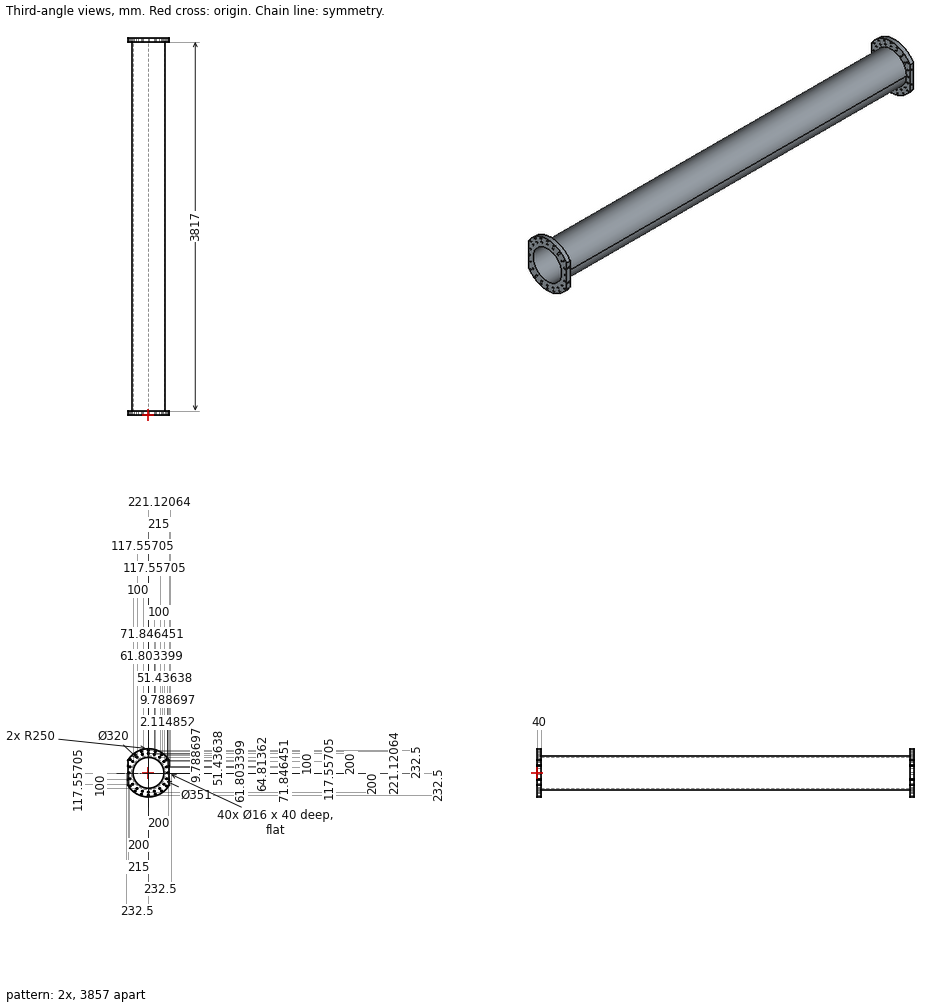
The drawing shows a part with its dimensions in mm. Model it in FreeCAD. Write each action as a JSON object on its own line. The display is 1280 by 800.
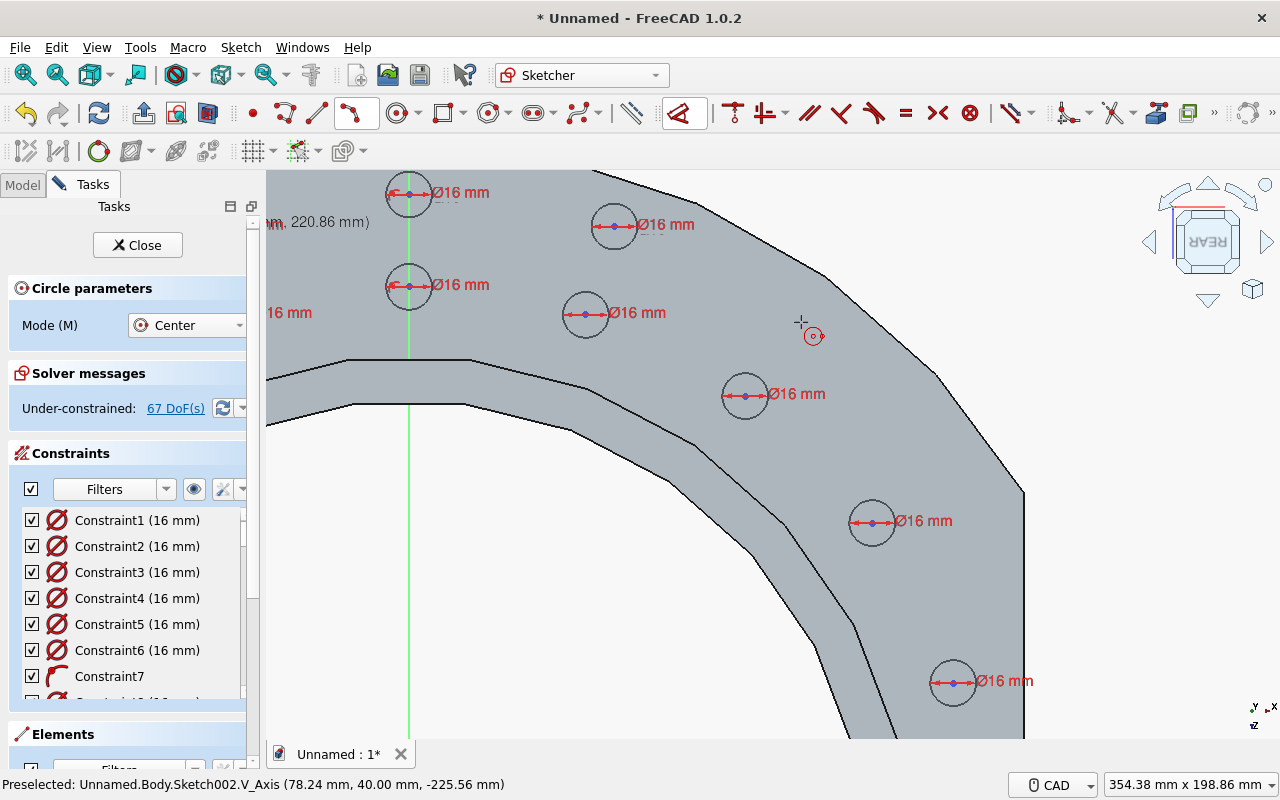
{"action": "left_click", "coordinate": [800, 320]}
{"action": "mouse_move", "coordinate": [816, 304]}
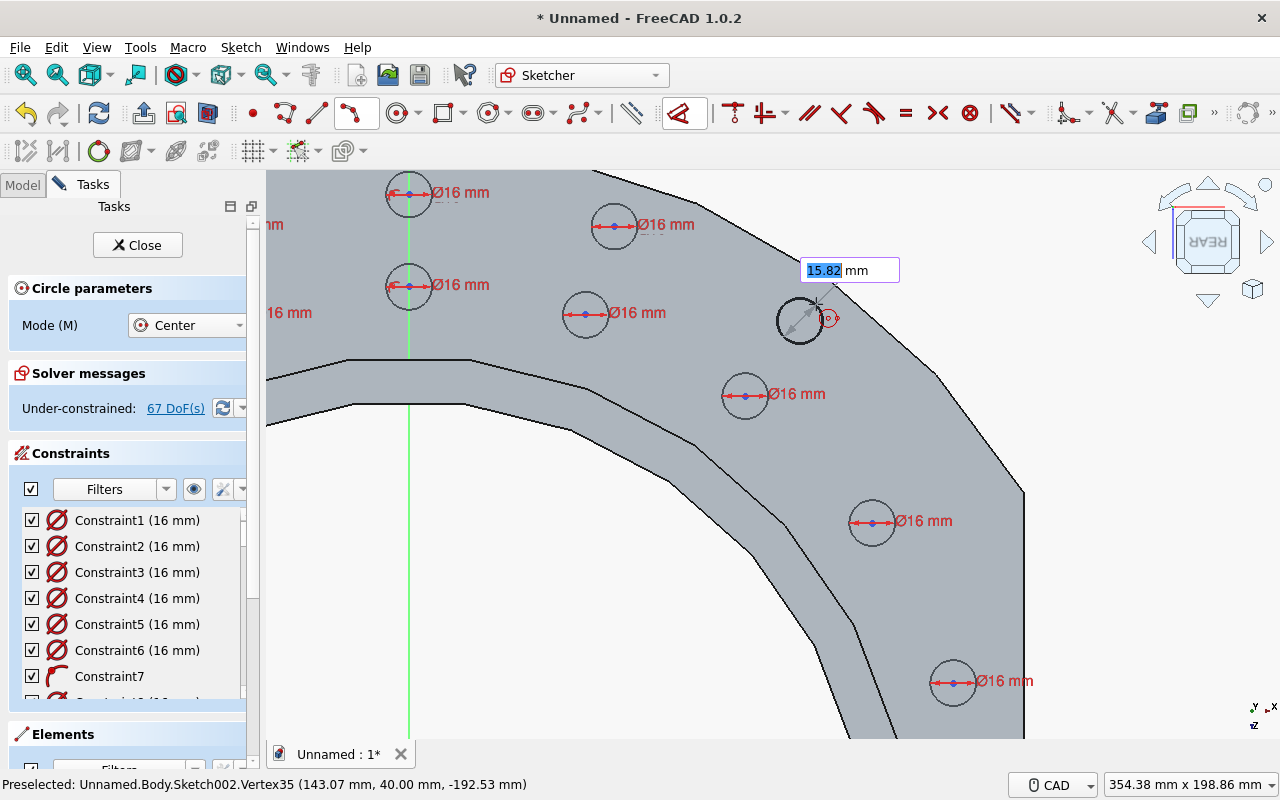
{"action": "type", "text": "16"}
{"action": "key", "text": "Return"}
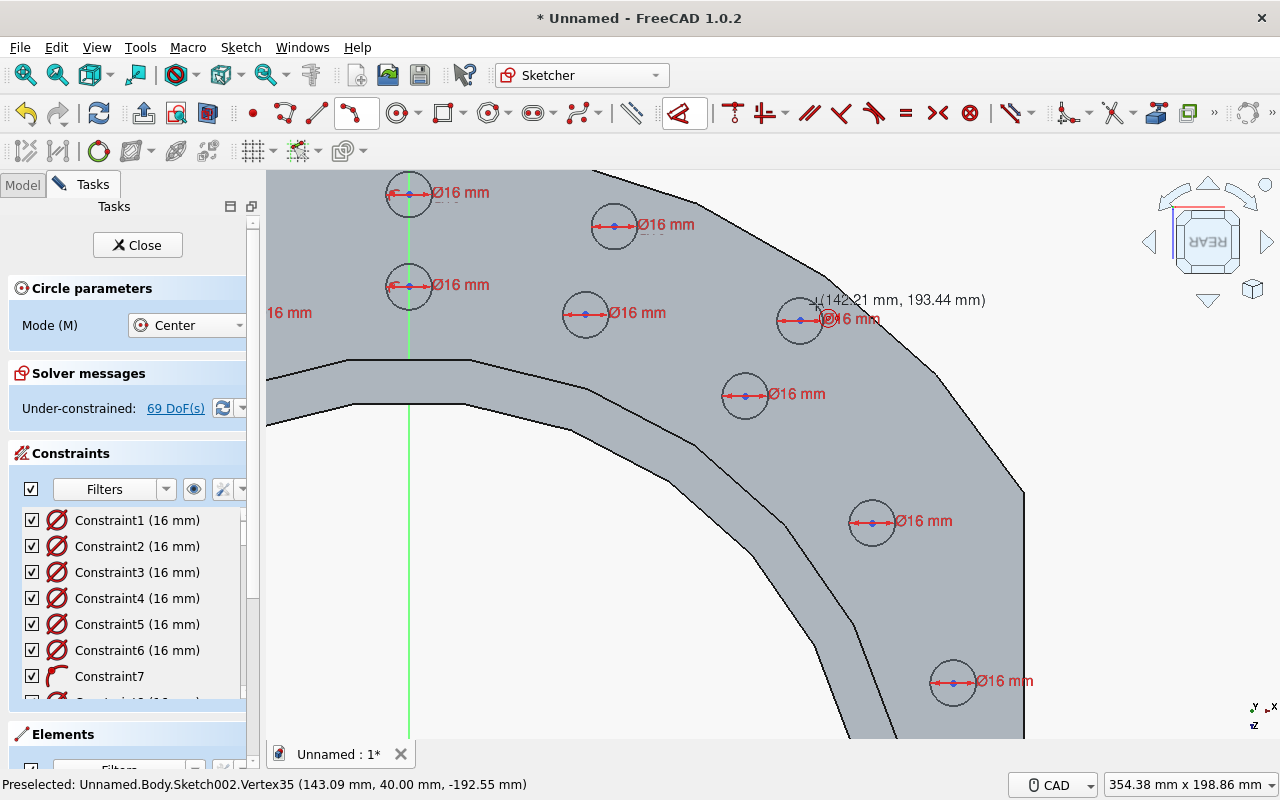
{"action": "left_click", "coordinate": [947, 467]}
{"action": "mouse_move", "coordinate": [963, 451]}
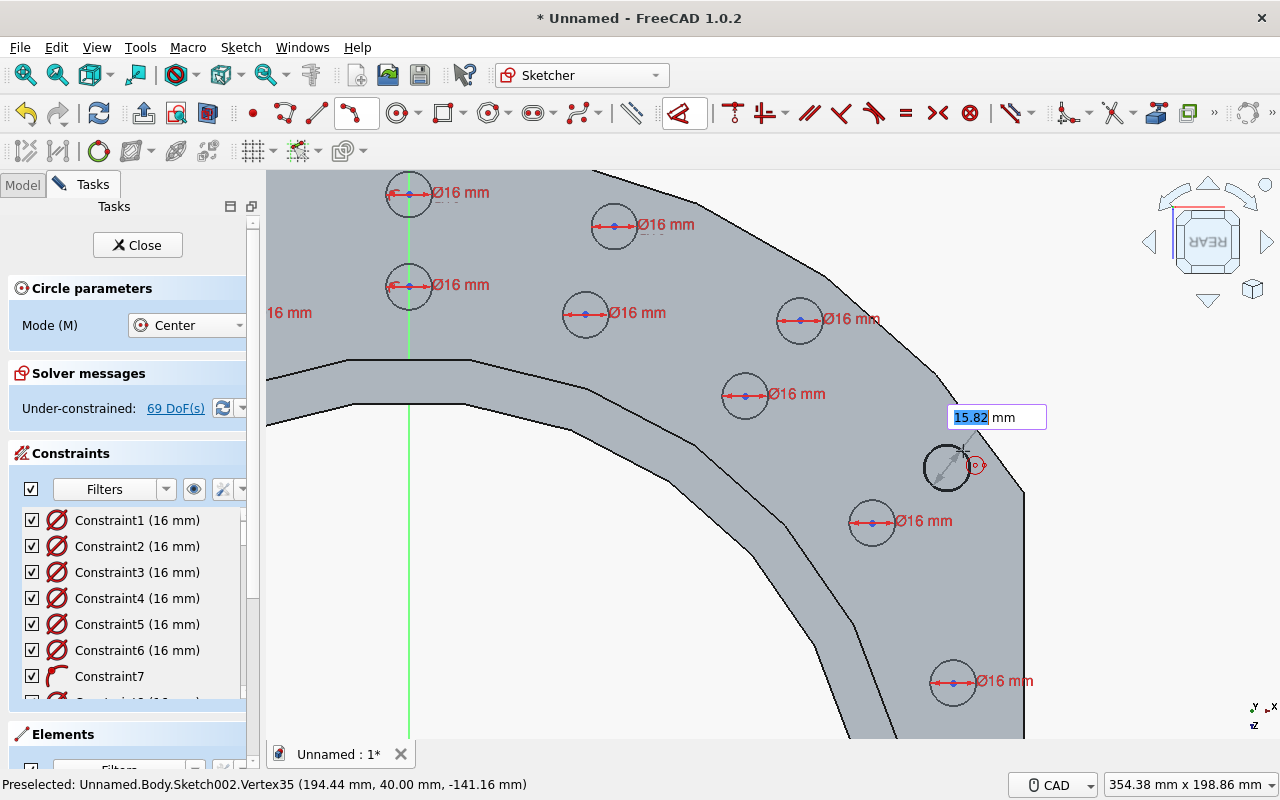
{"action": "type", "text": "16"}
{"action": "key", "text": "Return"}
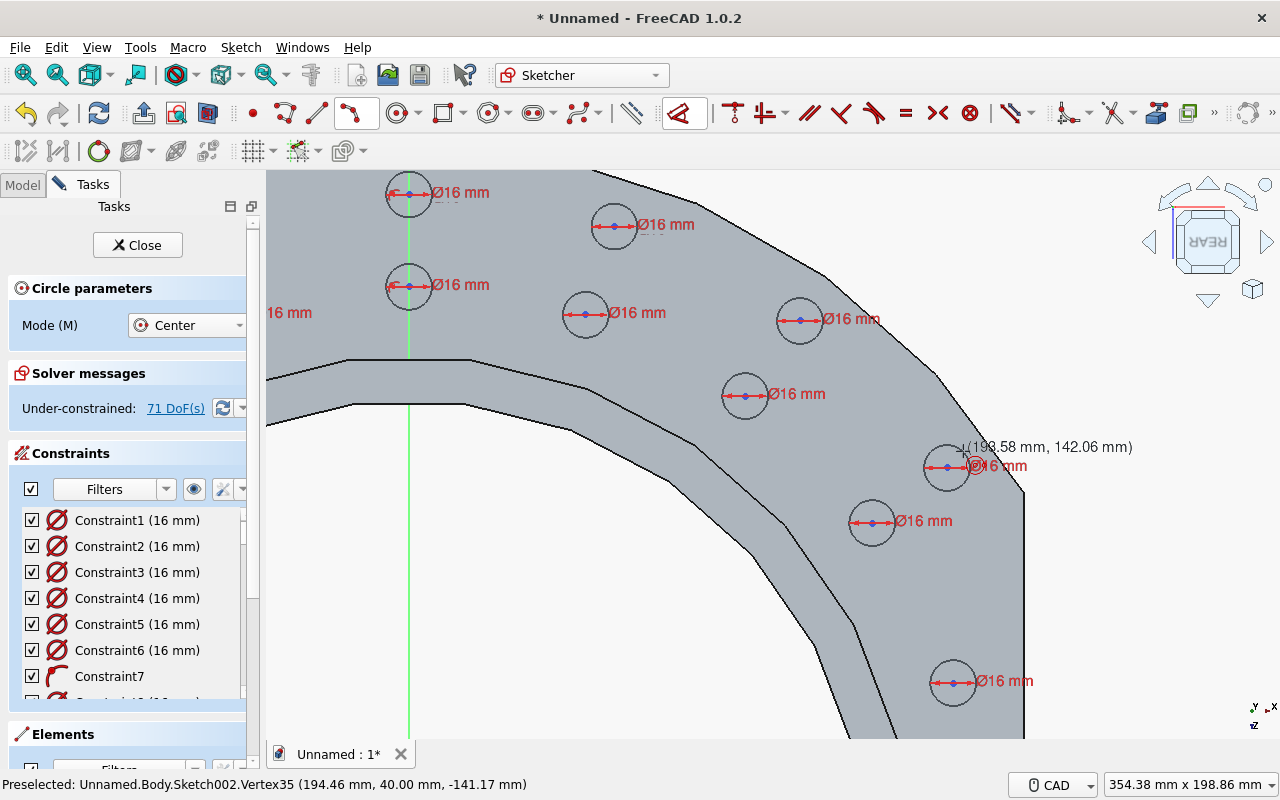
{"action": "left_click", "coordinate": [1042, 653]}
{"action": "mouse_move", "coordinate": [1058, 637]}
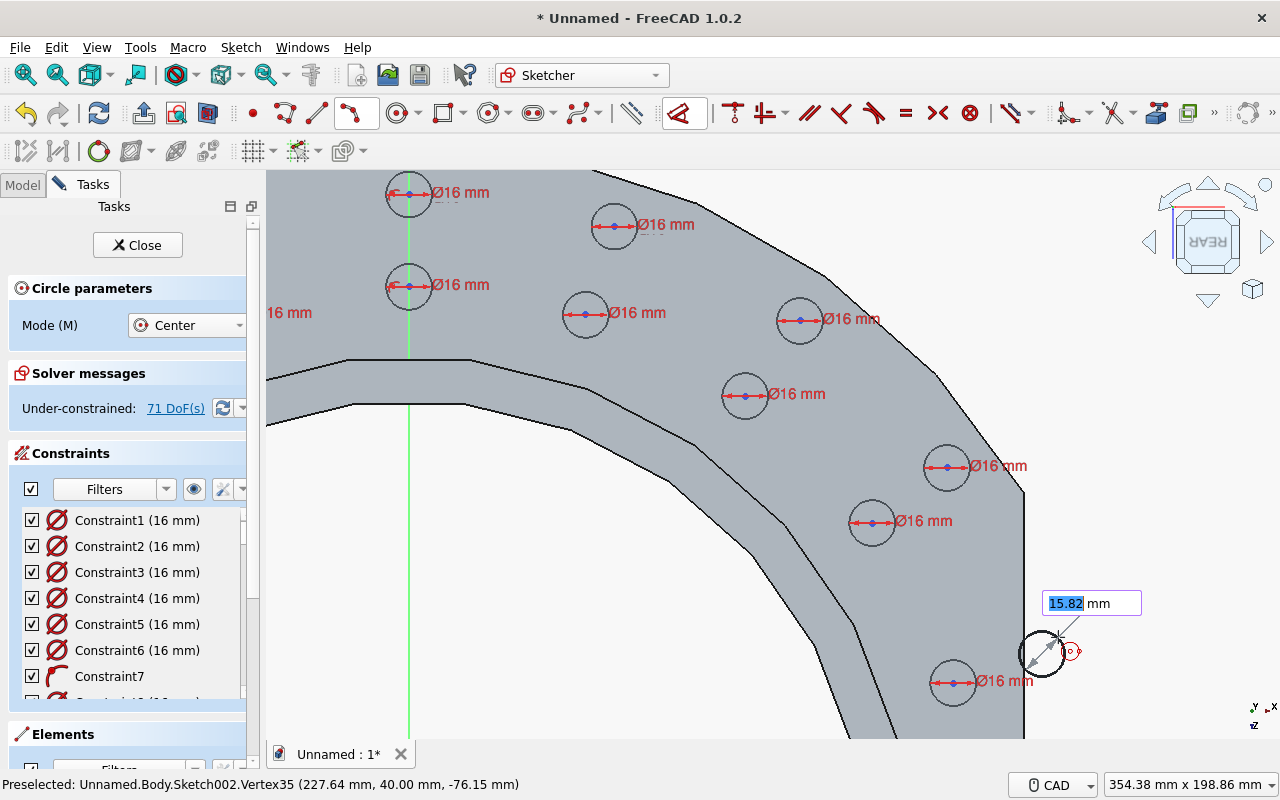
{"action": "type", "text": "16"}
{"action": "key", "text": "Return"}
{"action": "key", "text": "Escape"}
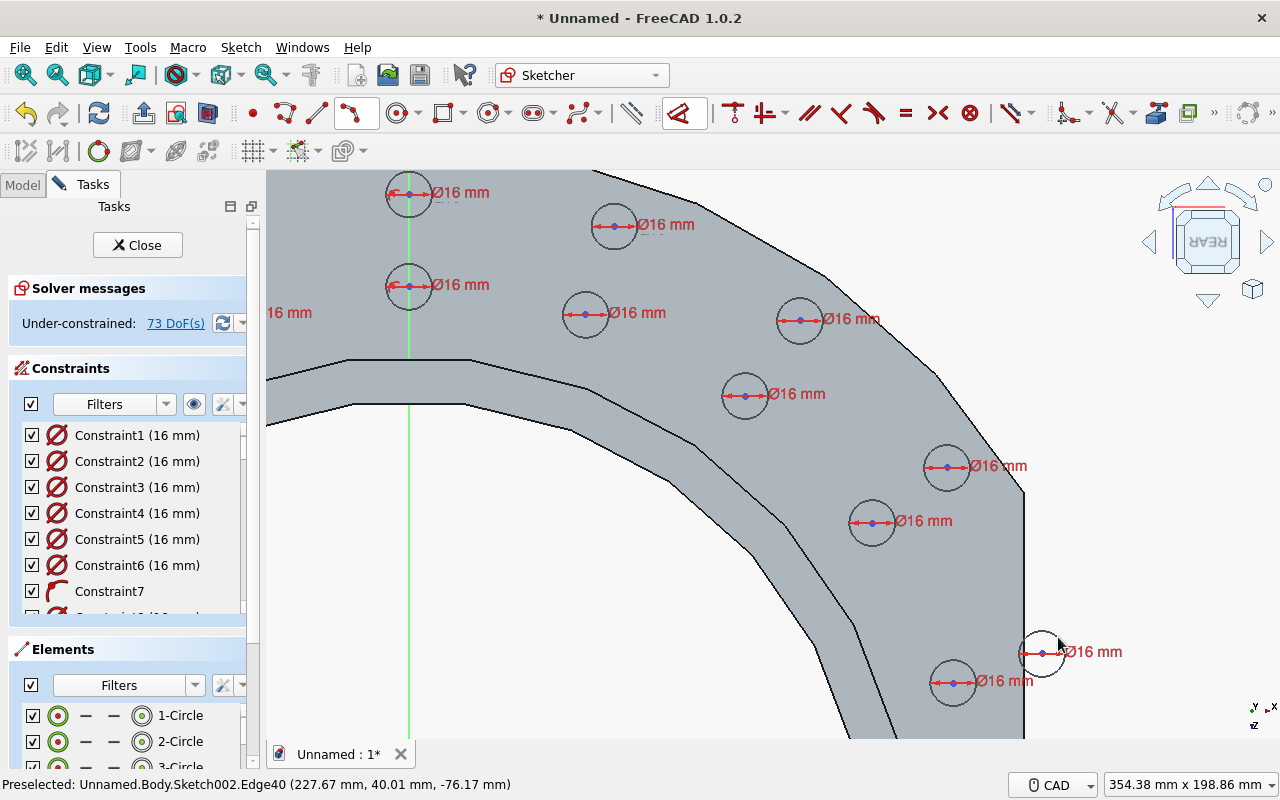
{"action": "scroll", "coordinate": [801, 322], "scroll_direction": "down", "scroll_amount": 7}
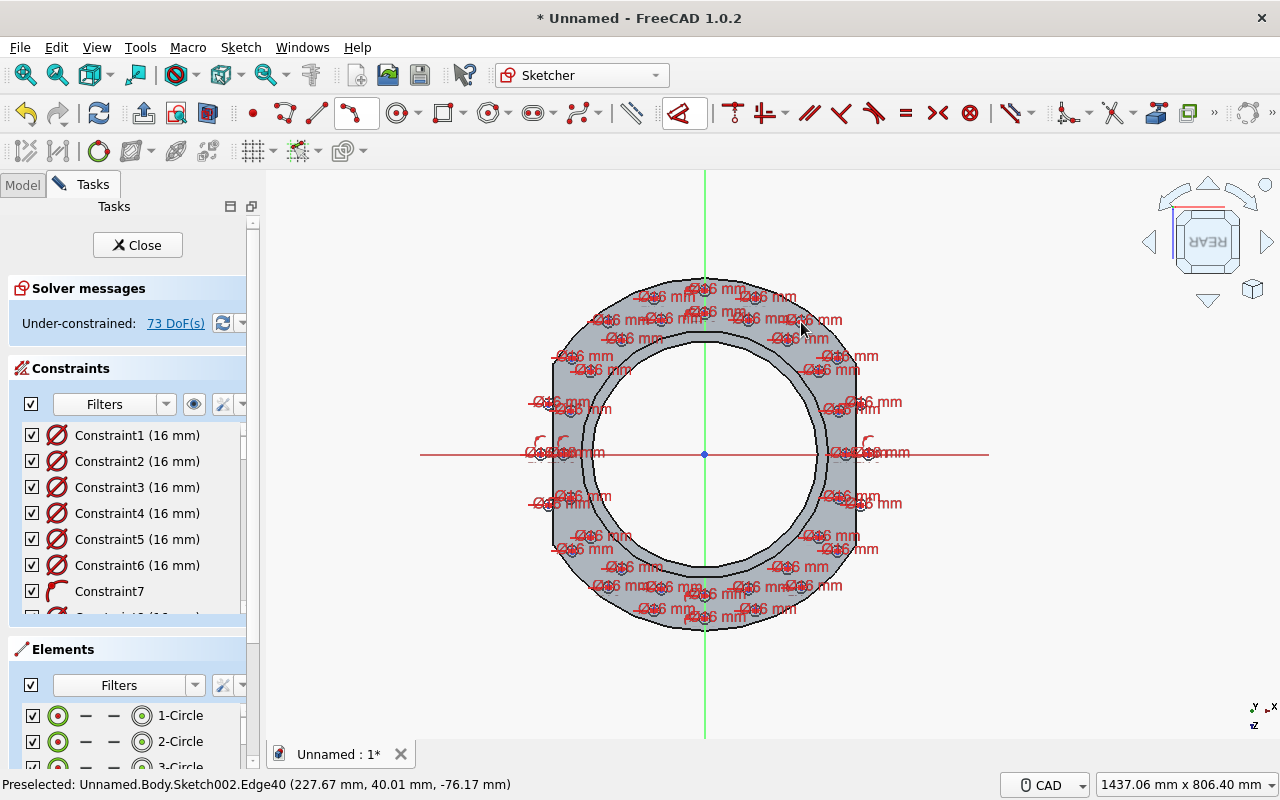
{"action": "left_click", "coordinate": [846, 455]}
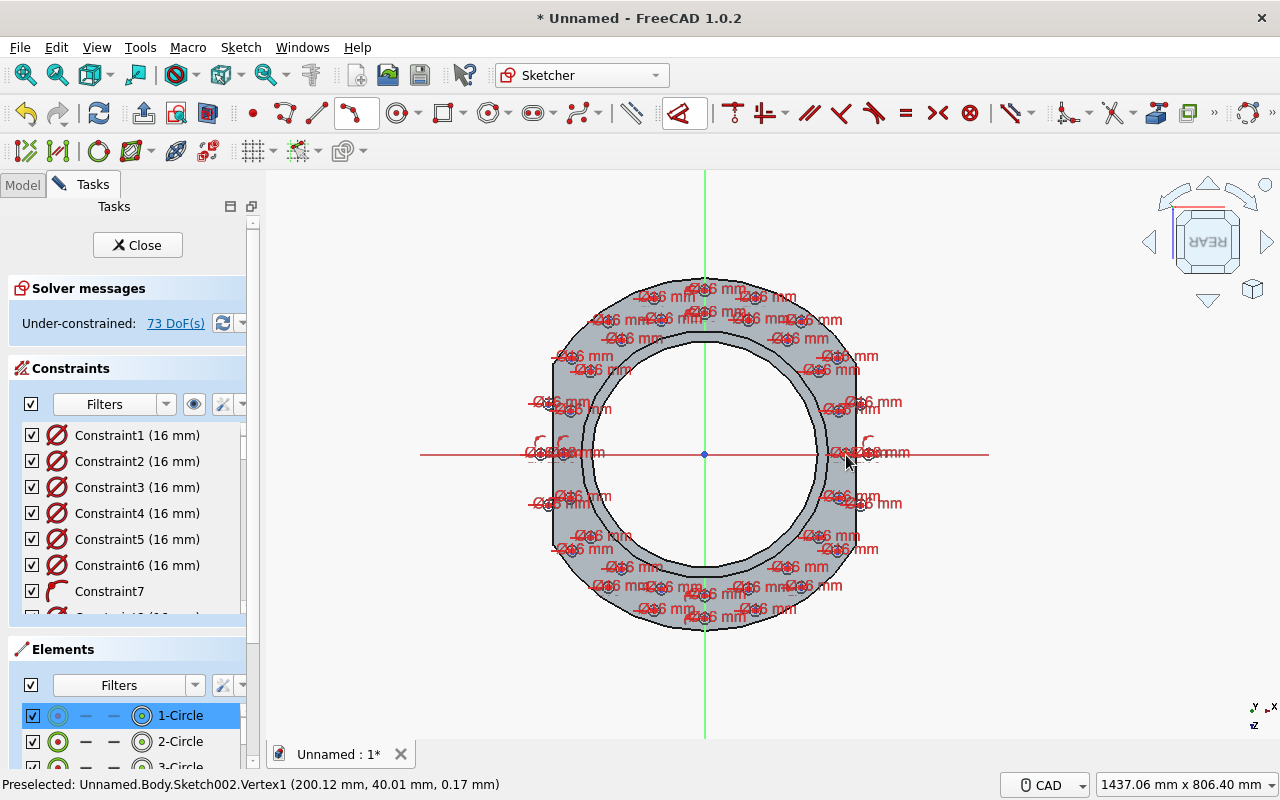
{"action": "left_click", "coordinate": [470, 454]}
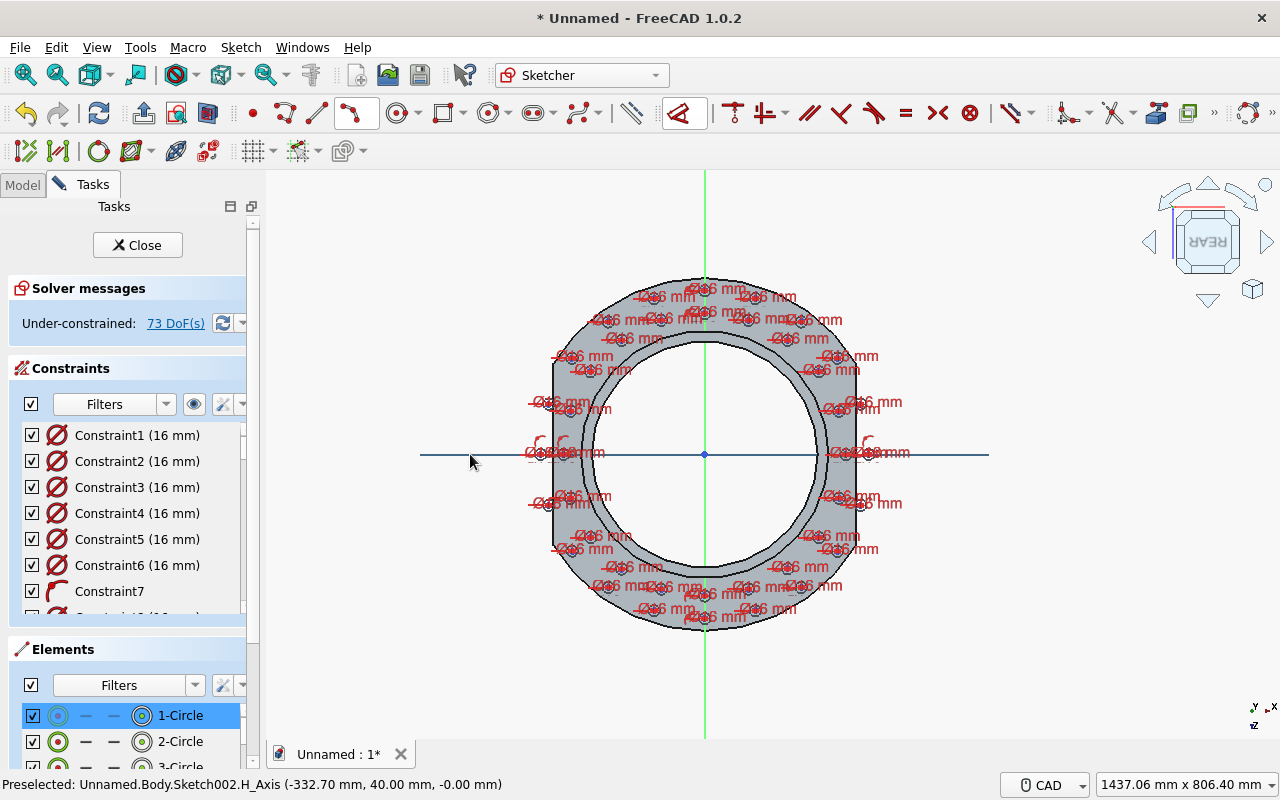
{"action": "key", "text": "c"}